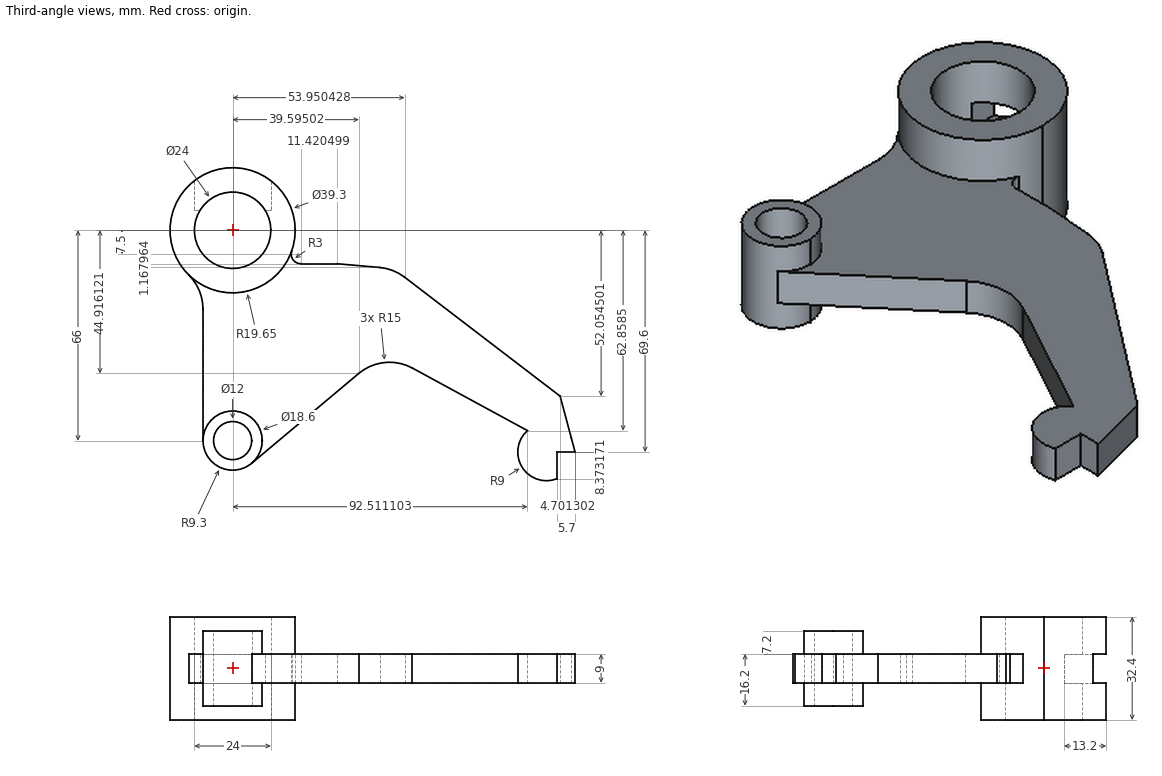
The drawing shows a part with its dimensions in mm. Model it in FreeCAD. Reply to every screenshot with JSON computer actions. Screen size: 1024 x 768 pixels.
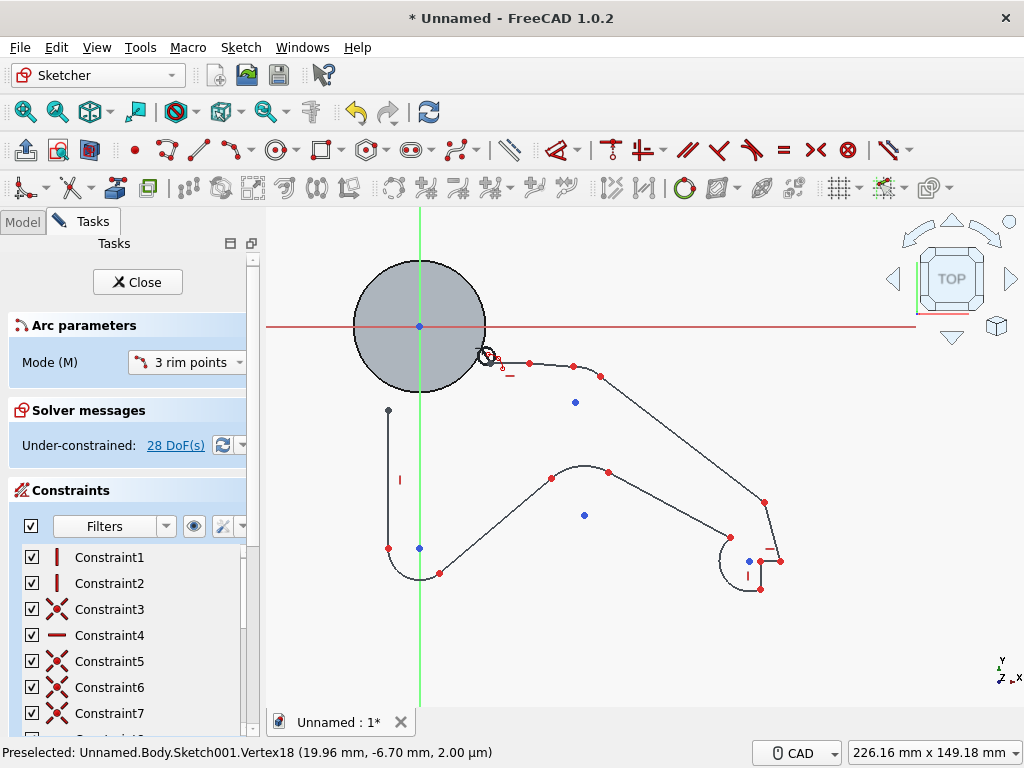
{"action": "scroll", "coordinate": [483, 357], "scroll_direction": "up", "scroll_amount": 7}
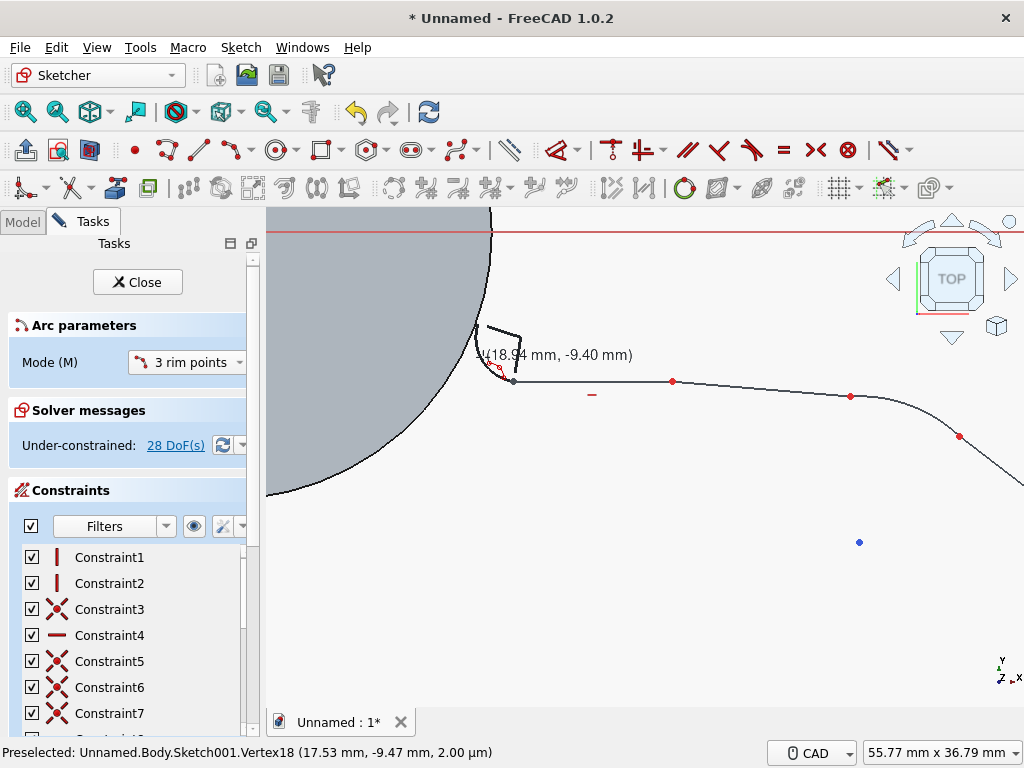
{"action": "left_click", "coordinate": [482, 358]}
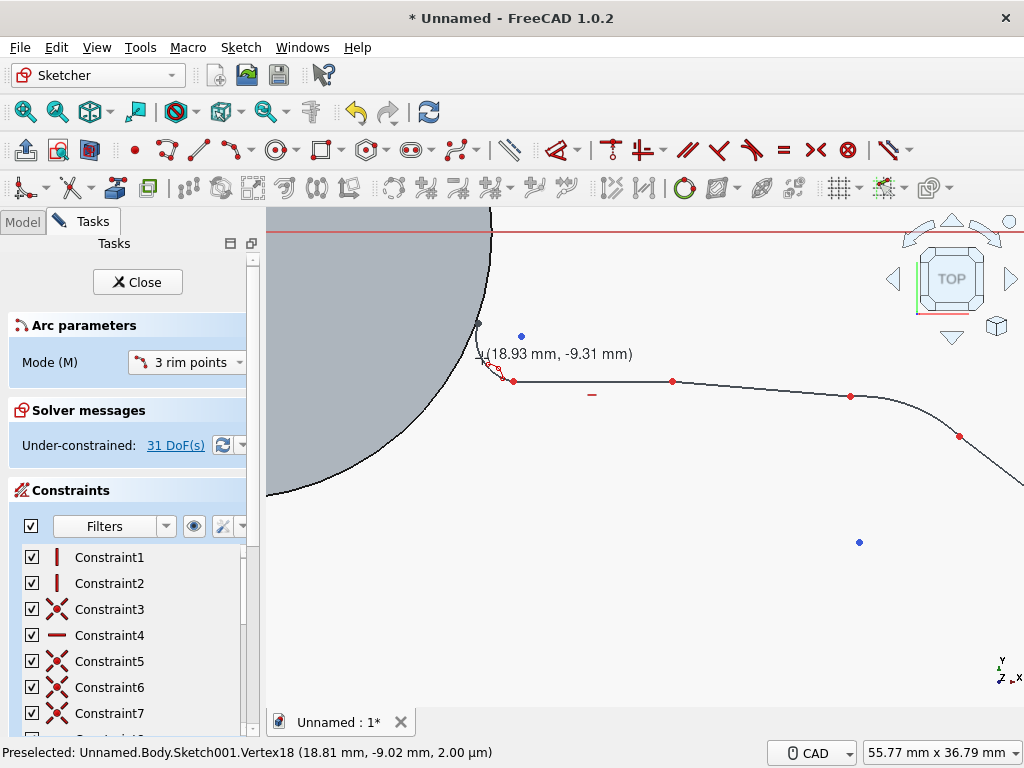
{"action": "left_click", "coordinate": [478, 324]}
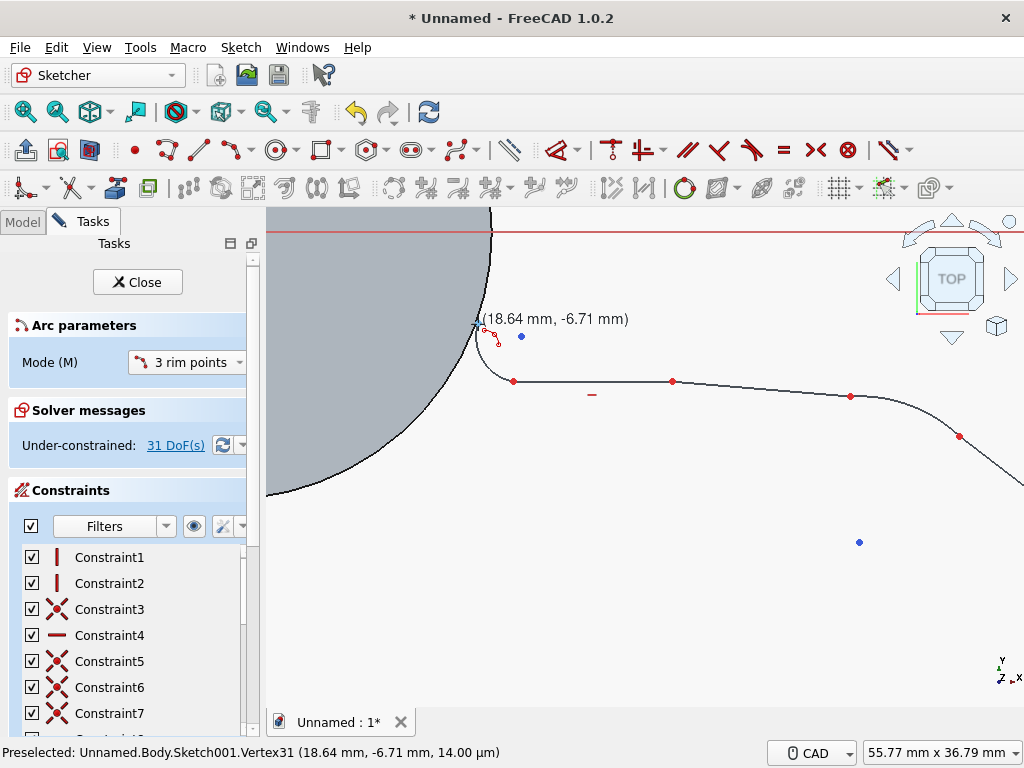
{"action": "scroll", "coordinate": [483, 357], "scroll_direction": "down", "scroll_amount": 7}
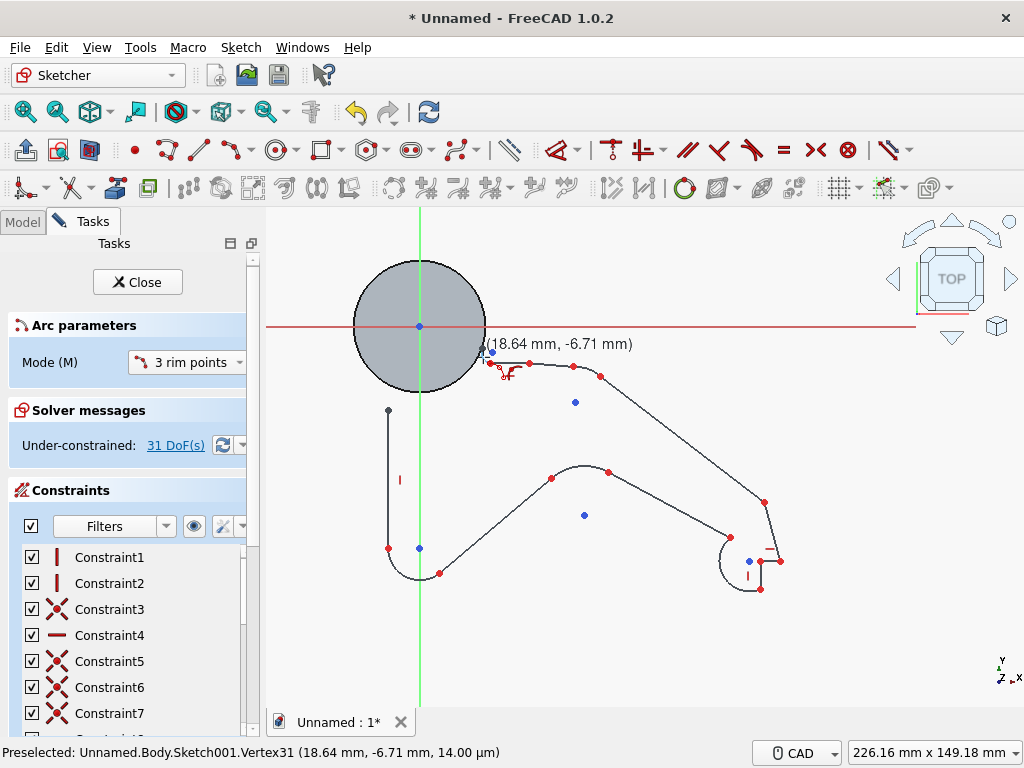
{"action": "left_click", "coordinate": [373, 373]}
{"action": "left_click", "coordinate": [447, 386]}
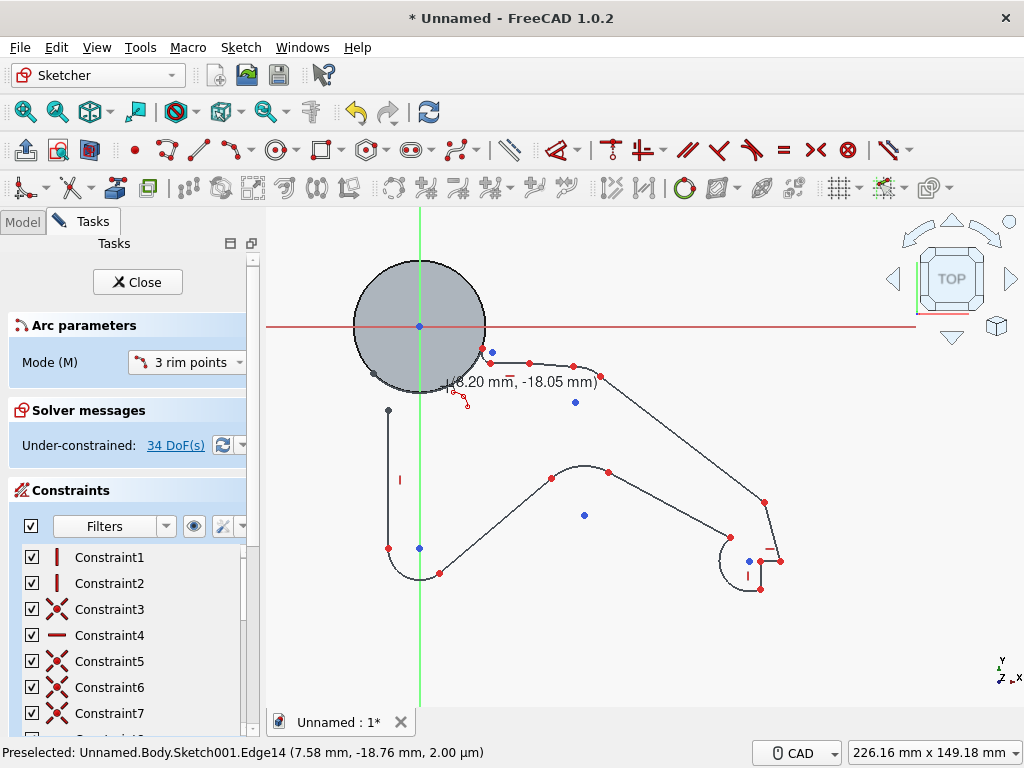
{"action": "left_click", "coordinate": [373, 374]}
{"action": "left_click", "coordinate": [388, 411]}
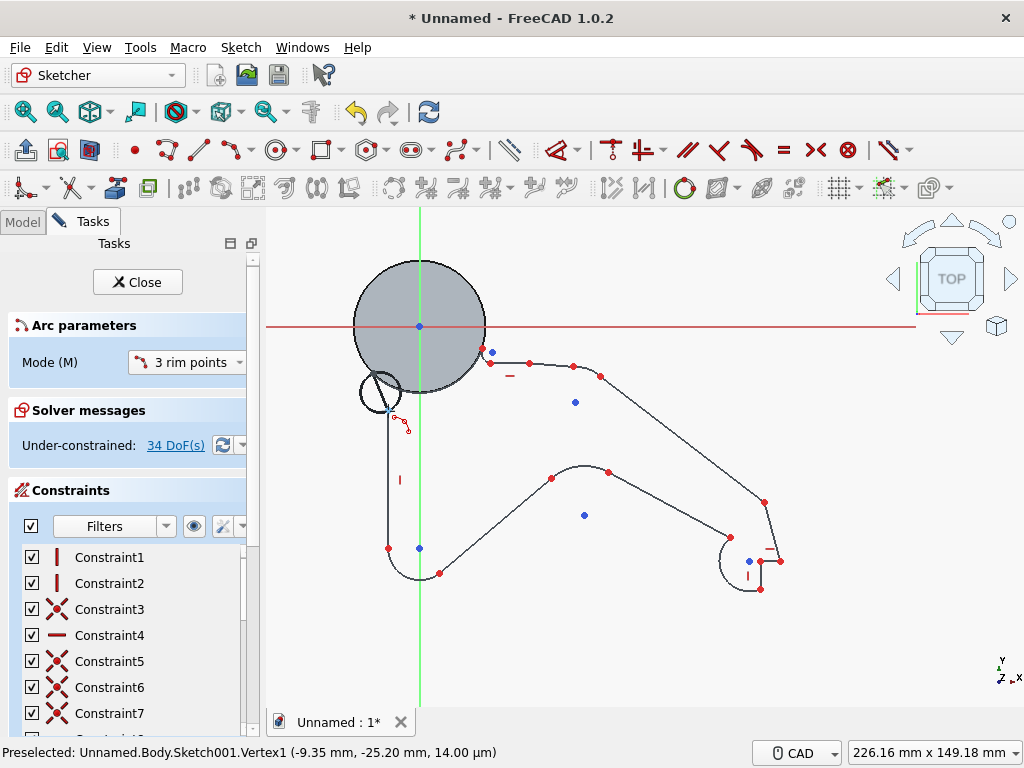
{"action": "scroll", "coordinate": [384, 390], "scroll_direction": "up", "scroll_amount": 8}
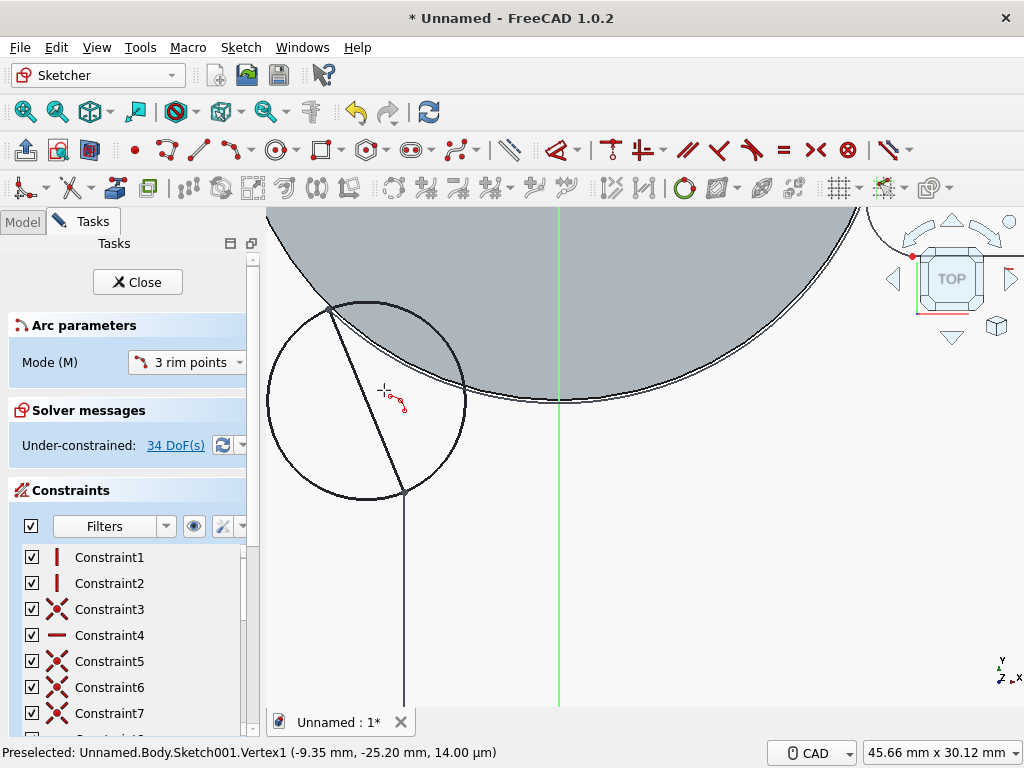
{"action": "left_click", "coordinate": [386, 388]}
{"action": "key", "text": "Escape"}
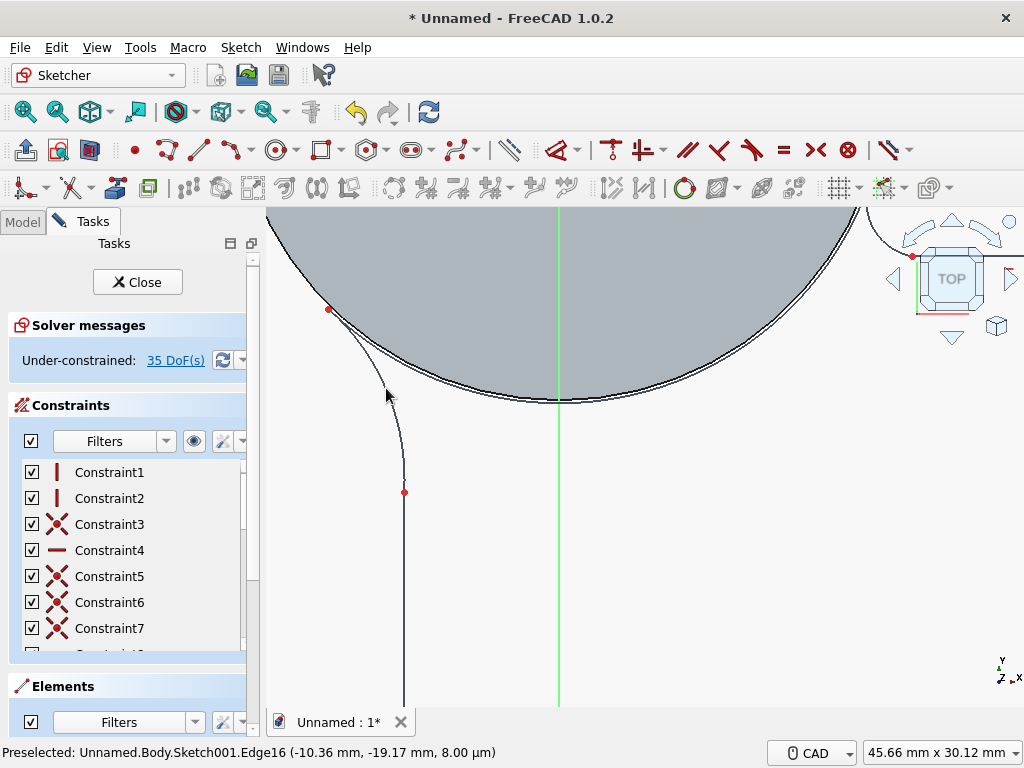
{"action": "scroll", "coordinate": [384, 390], "scroll_direction": "down", "scroll_amount": 8}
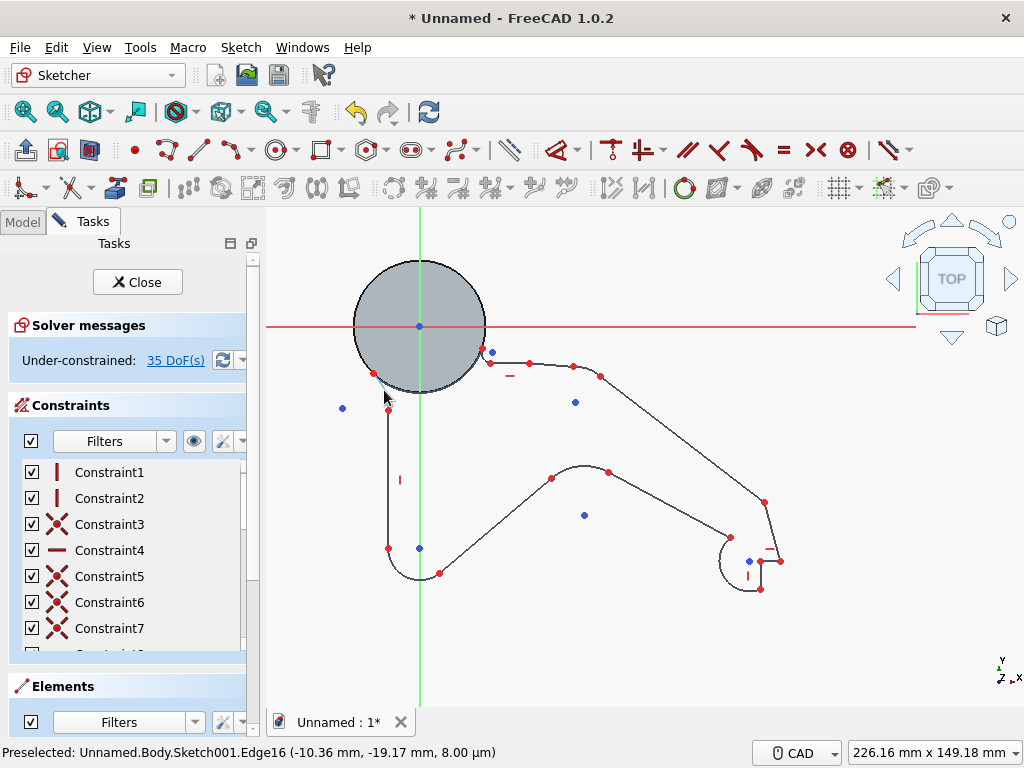
{"action": "left_click", "coordinate": [388, 439]}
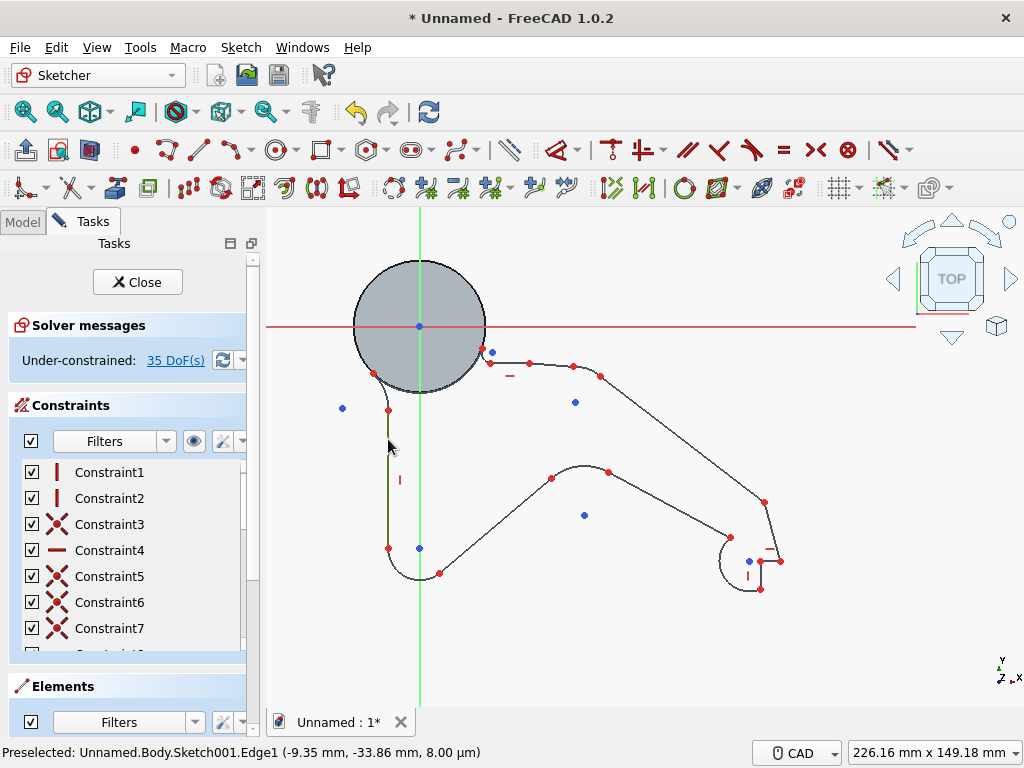
{"action": "left_click", "coordinate": [395, 568]}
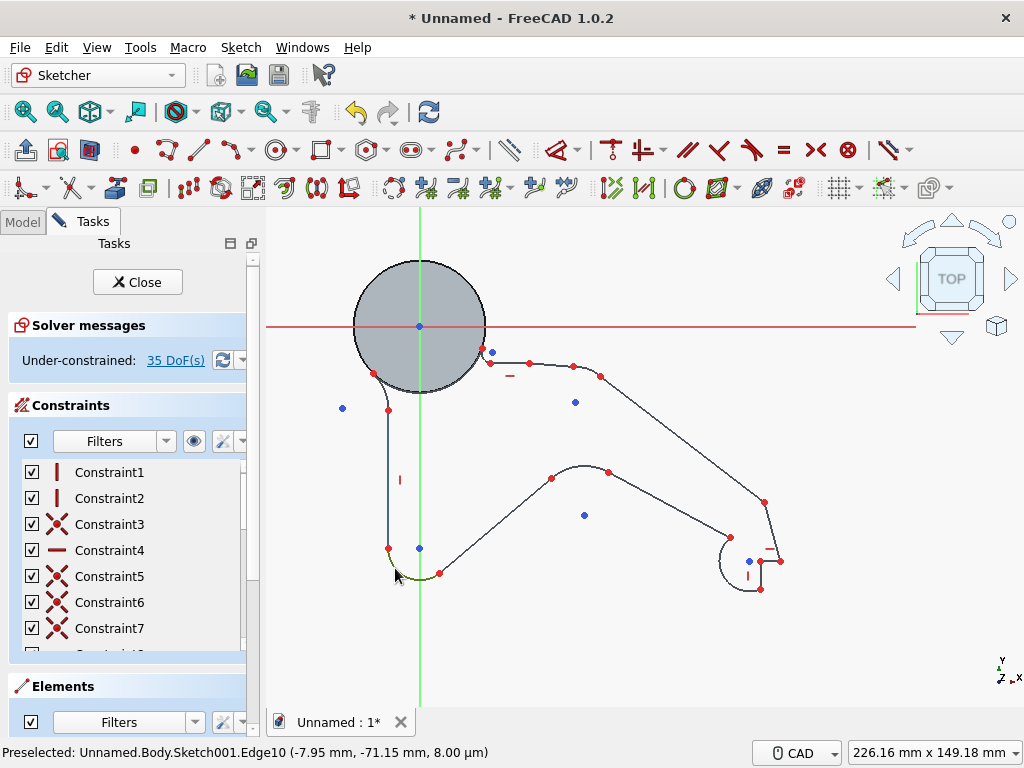
{"action": "key", "text": "t"}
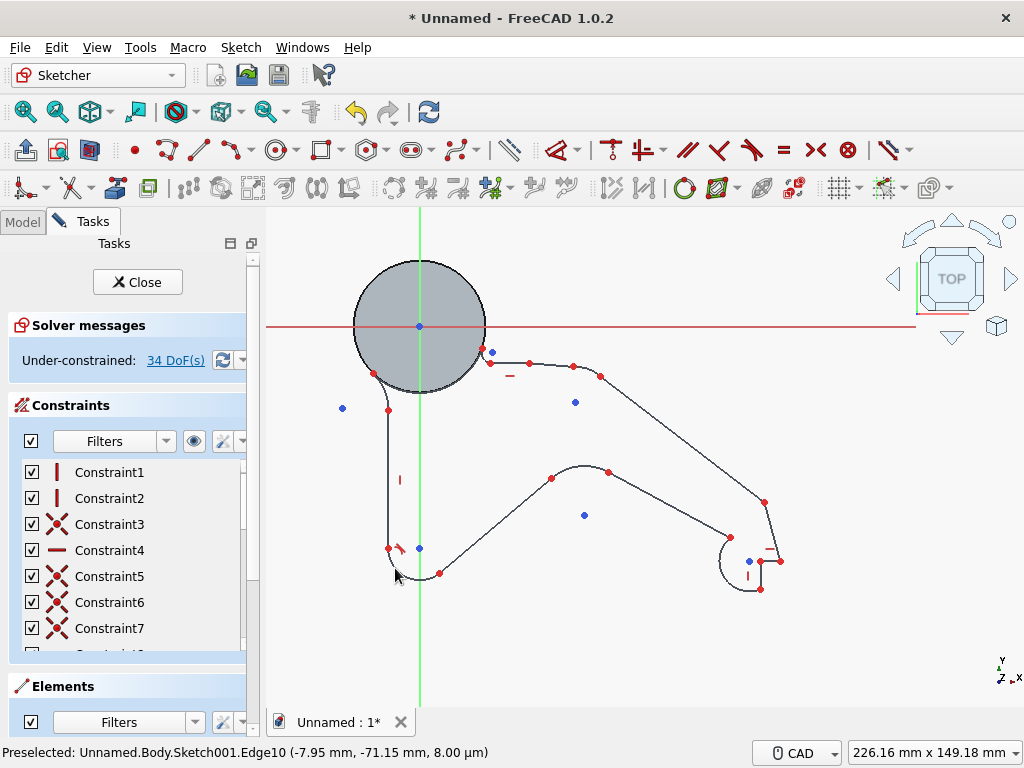
{"action": "left_click", "coordinate": [388, 452]}